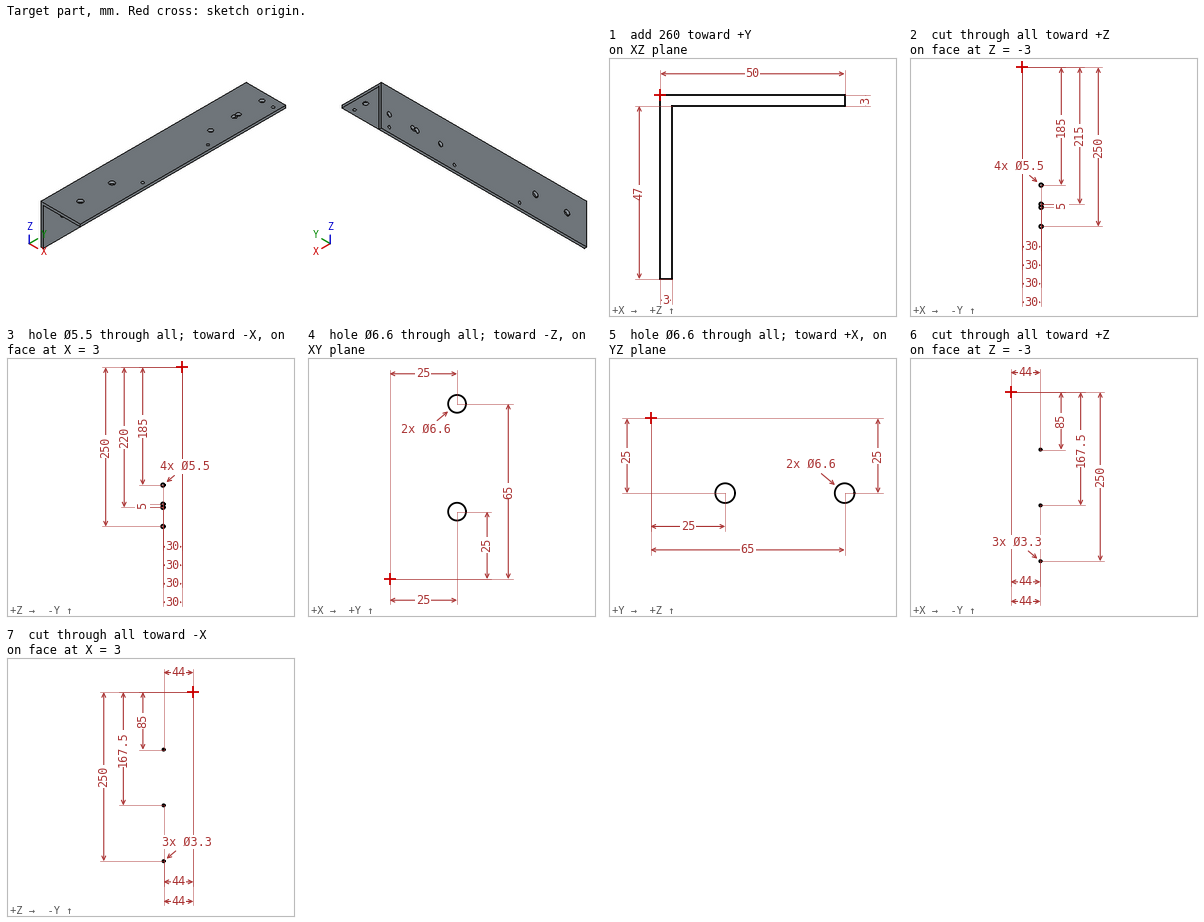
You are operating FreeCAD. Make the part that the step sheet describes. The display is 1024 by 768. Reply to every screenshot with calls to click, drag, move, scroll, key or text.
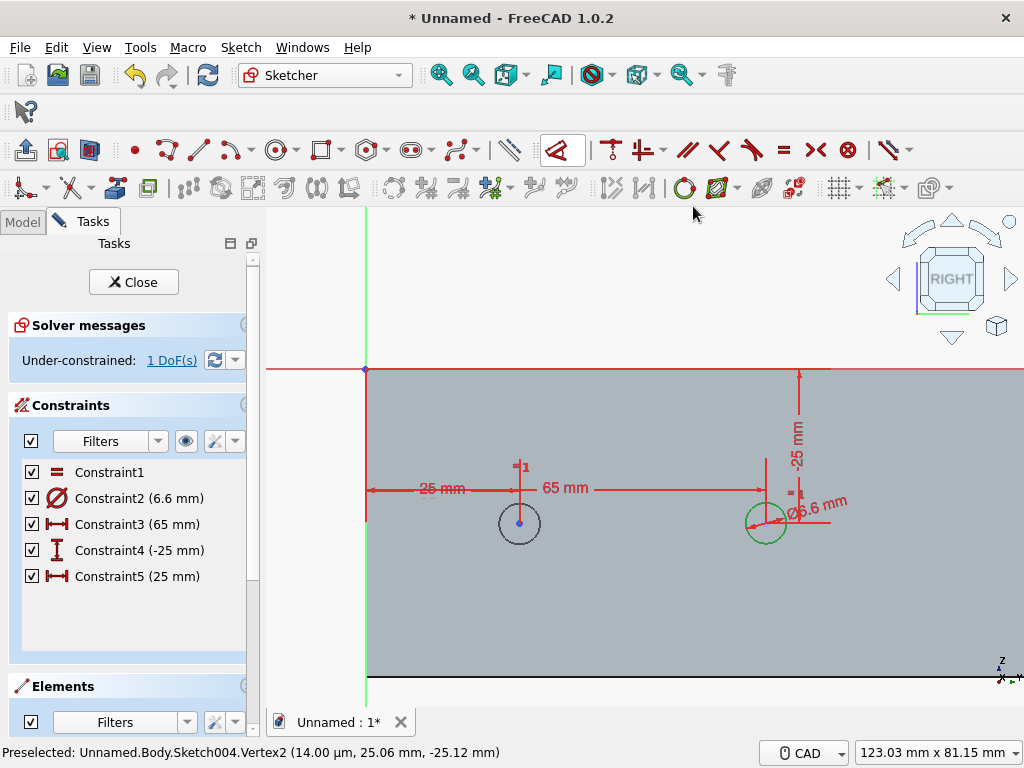
click(520, 524)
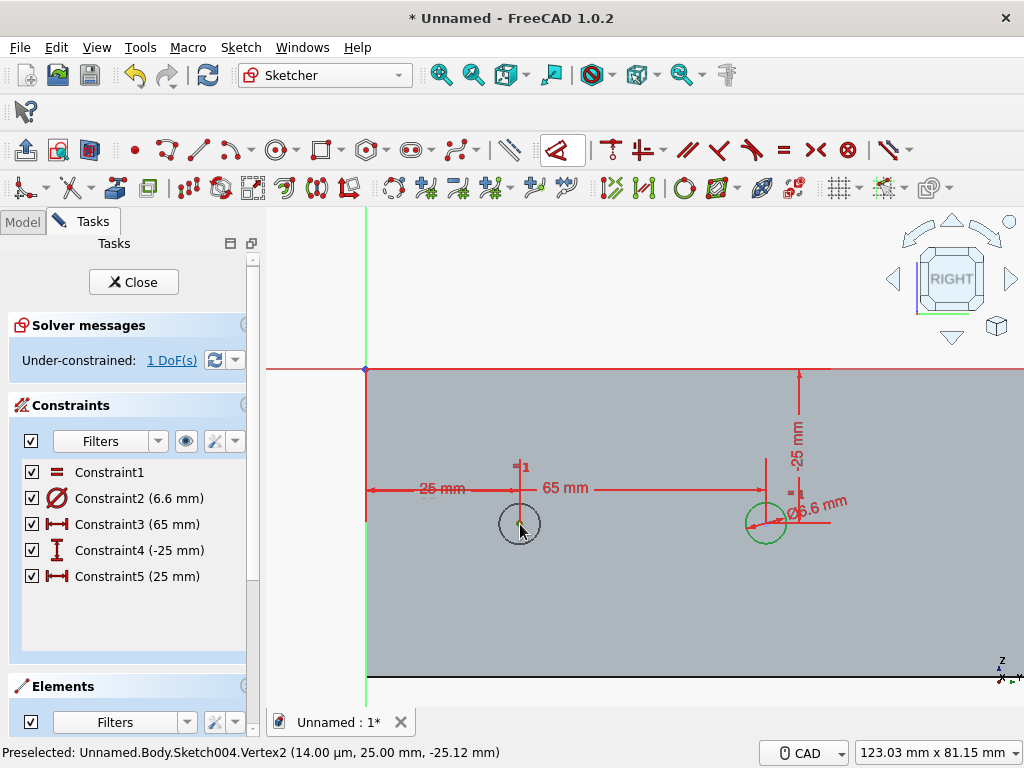
click(580, 150)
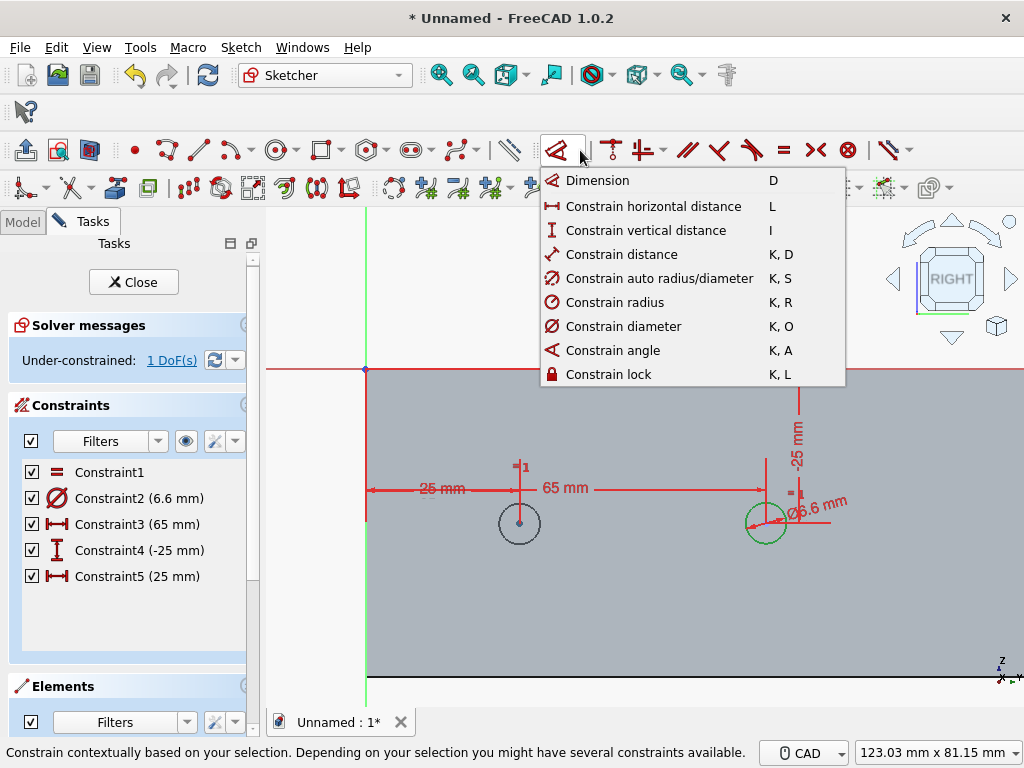
click(693, 230)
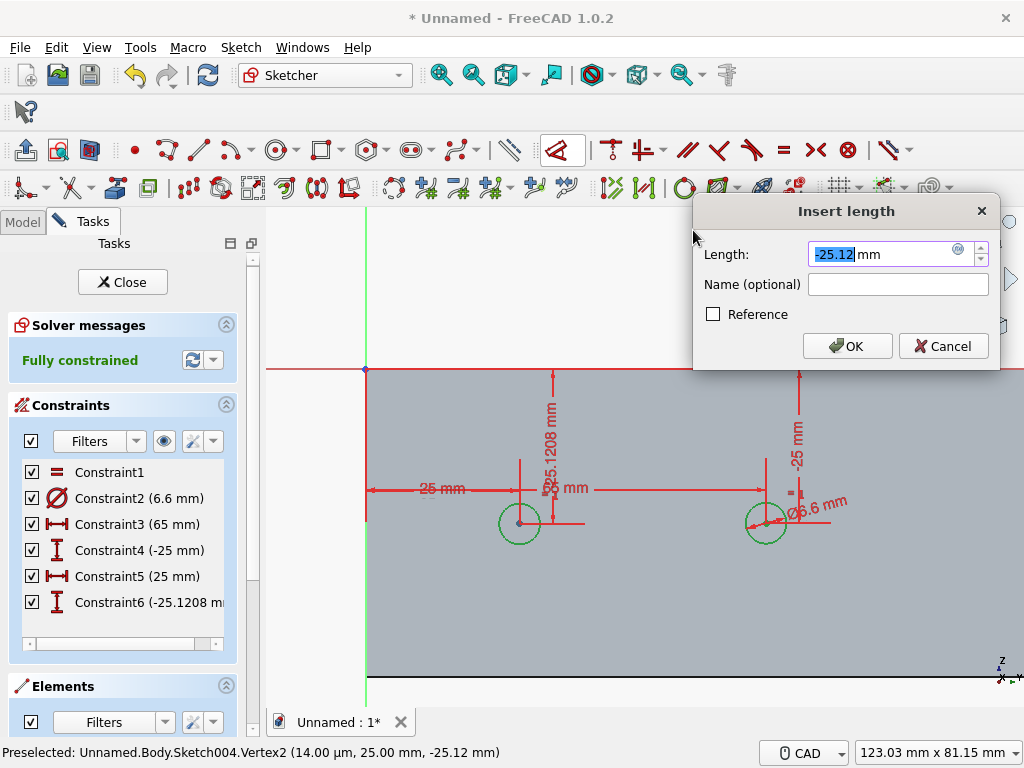
text(-25)
key(Return)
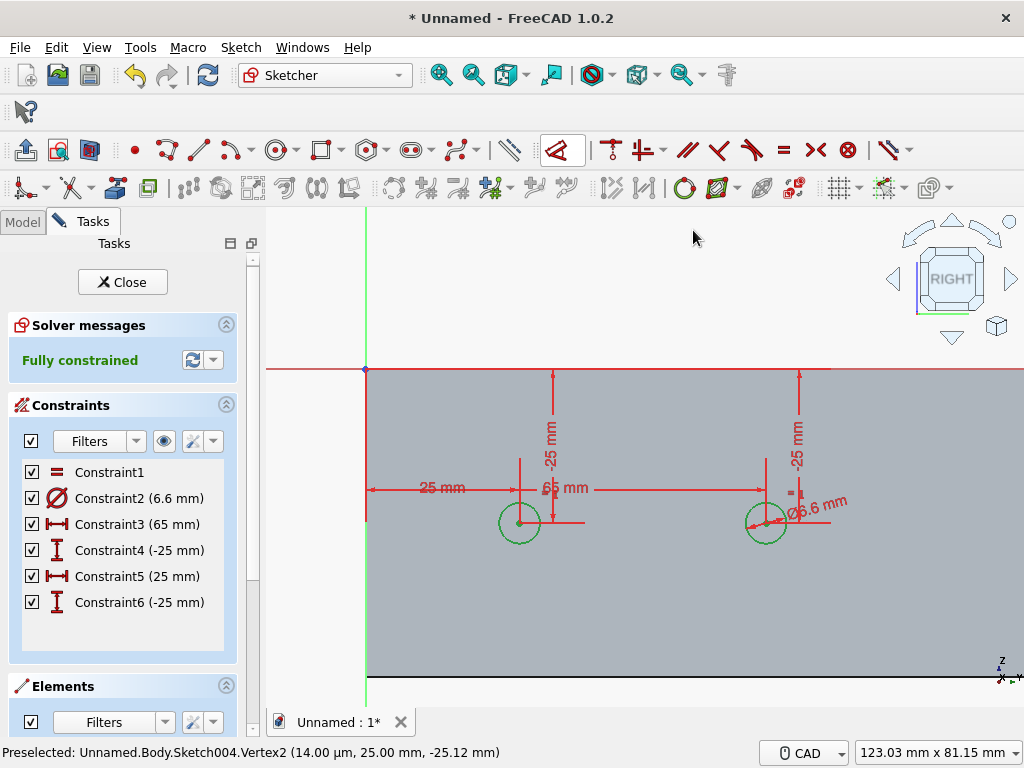
click(123, 282)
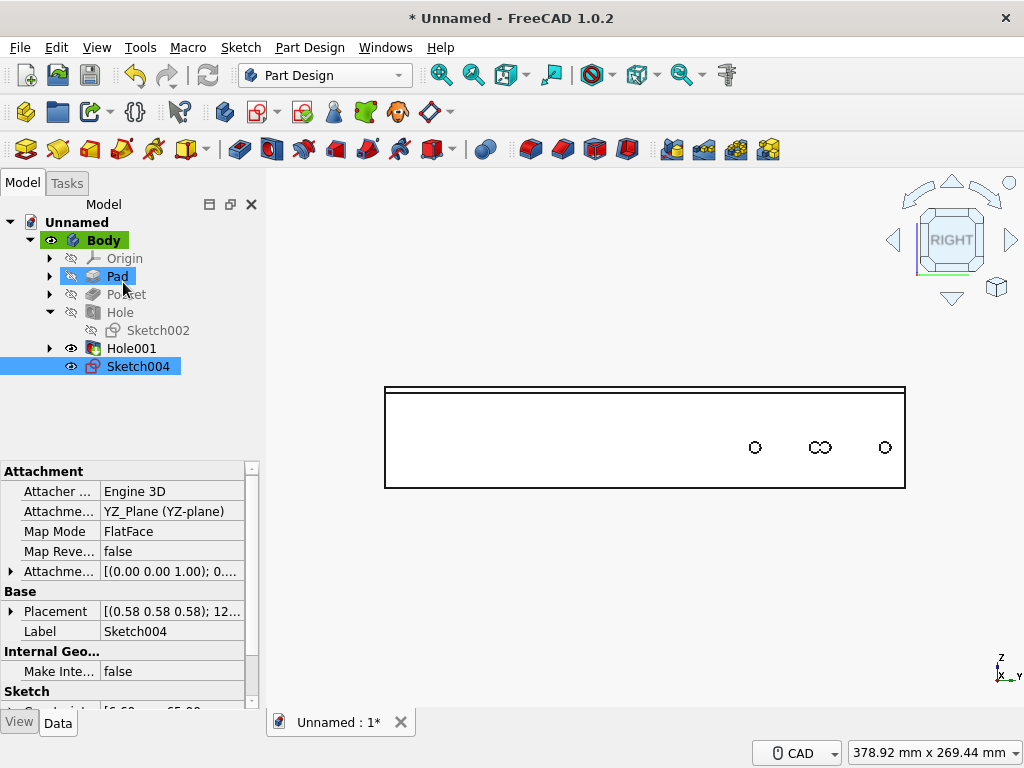
click(272, 150)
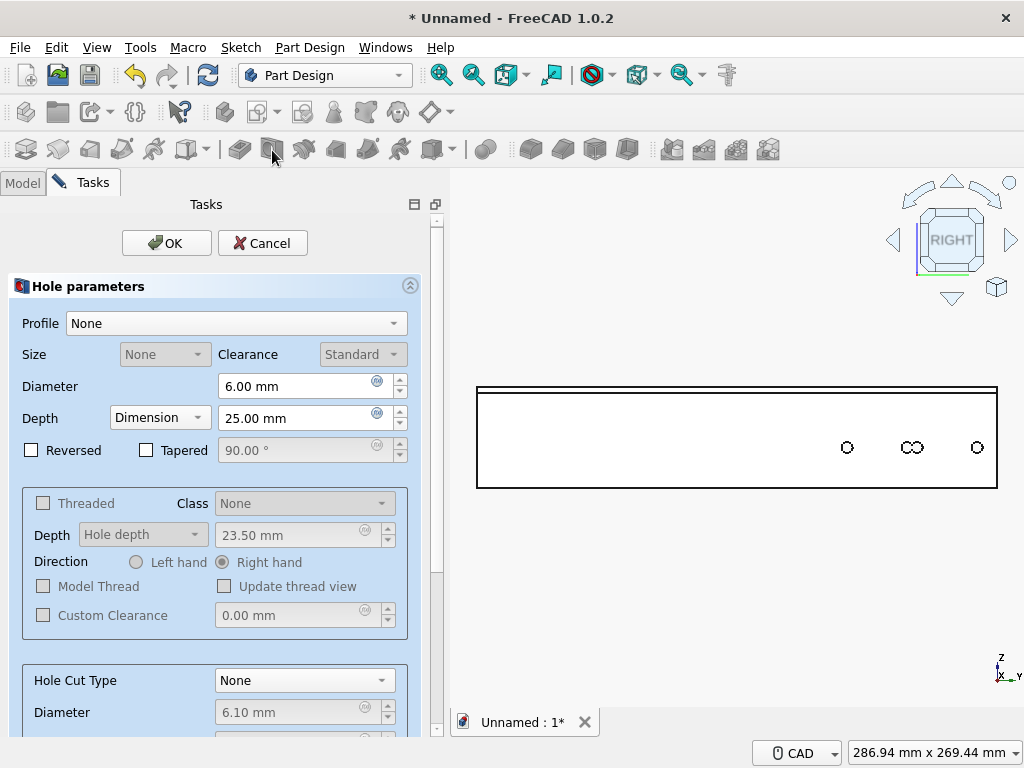
triple_click(305, 386)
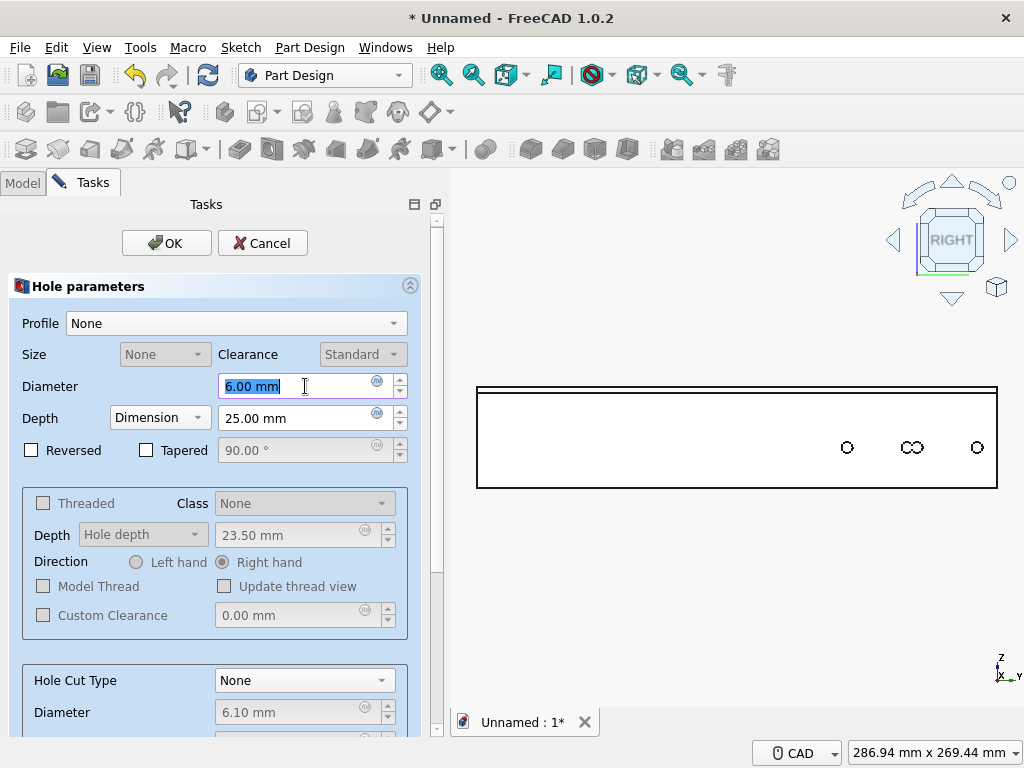
text(6.6)
key(Tab)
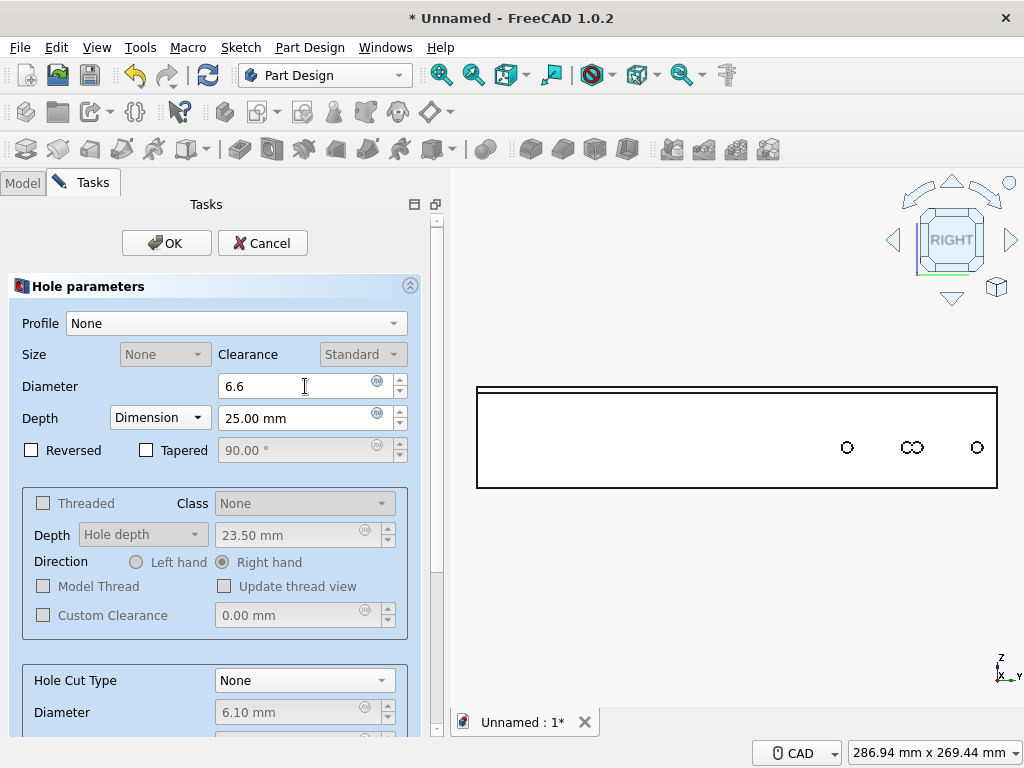
click(161, 418)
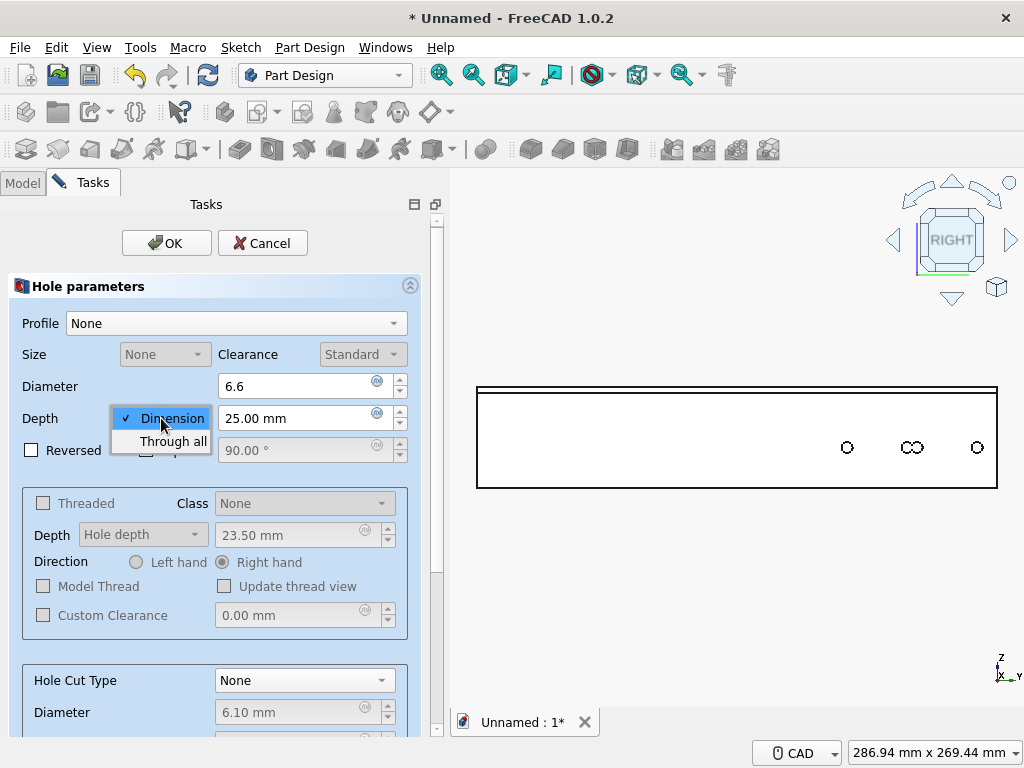
click(160, 442)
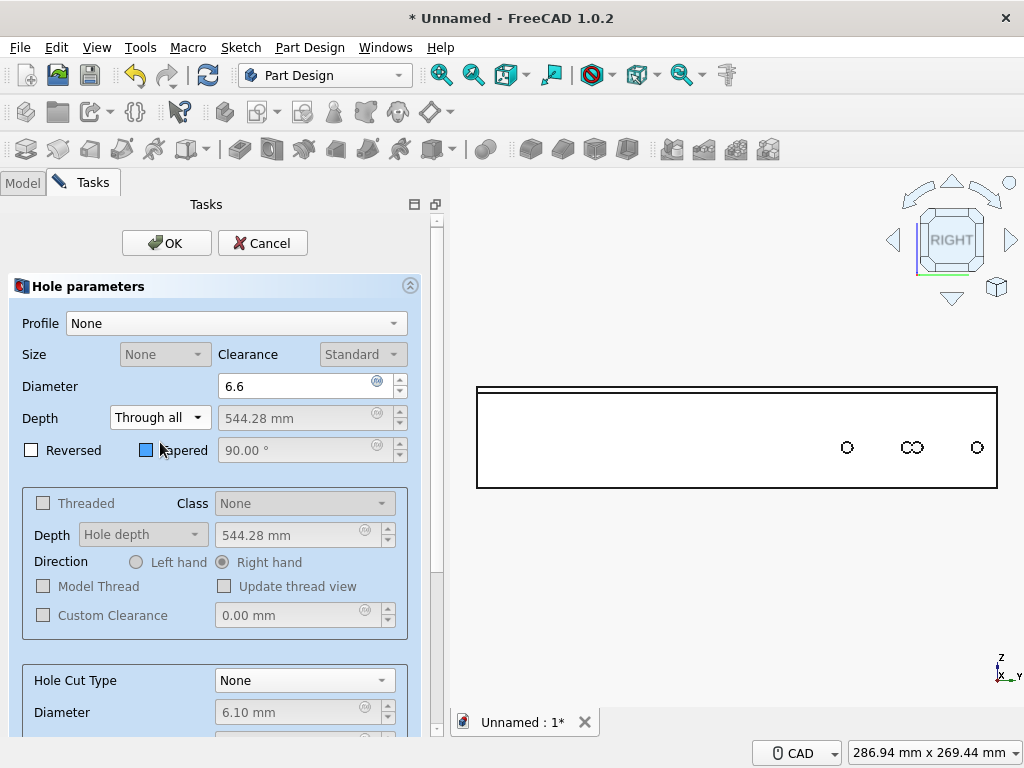
click(30, 450)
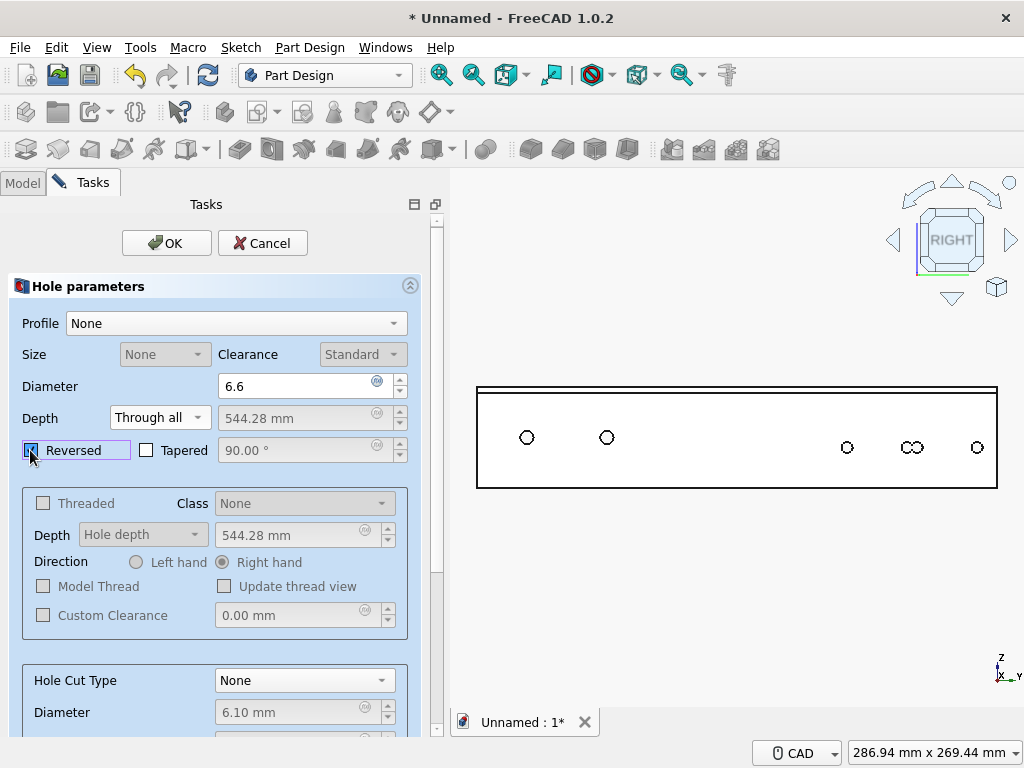
click(167, 243)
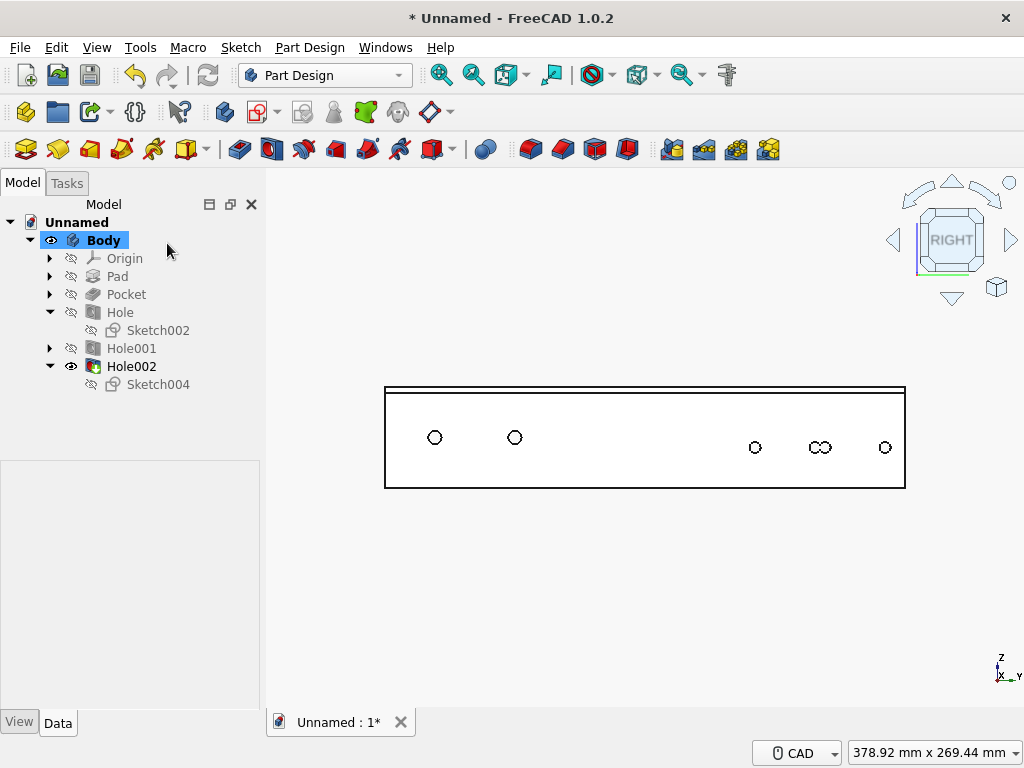
key(5)